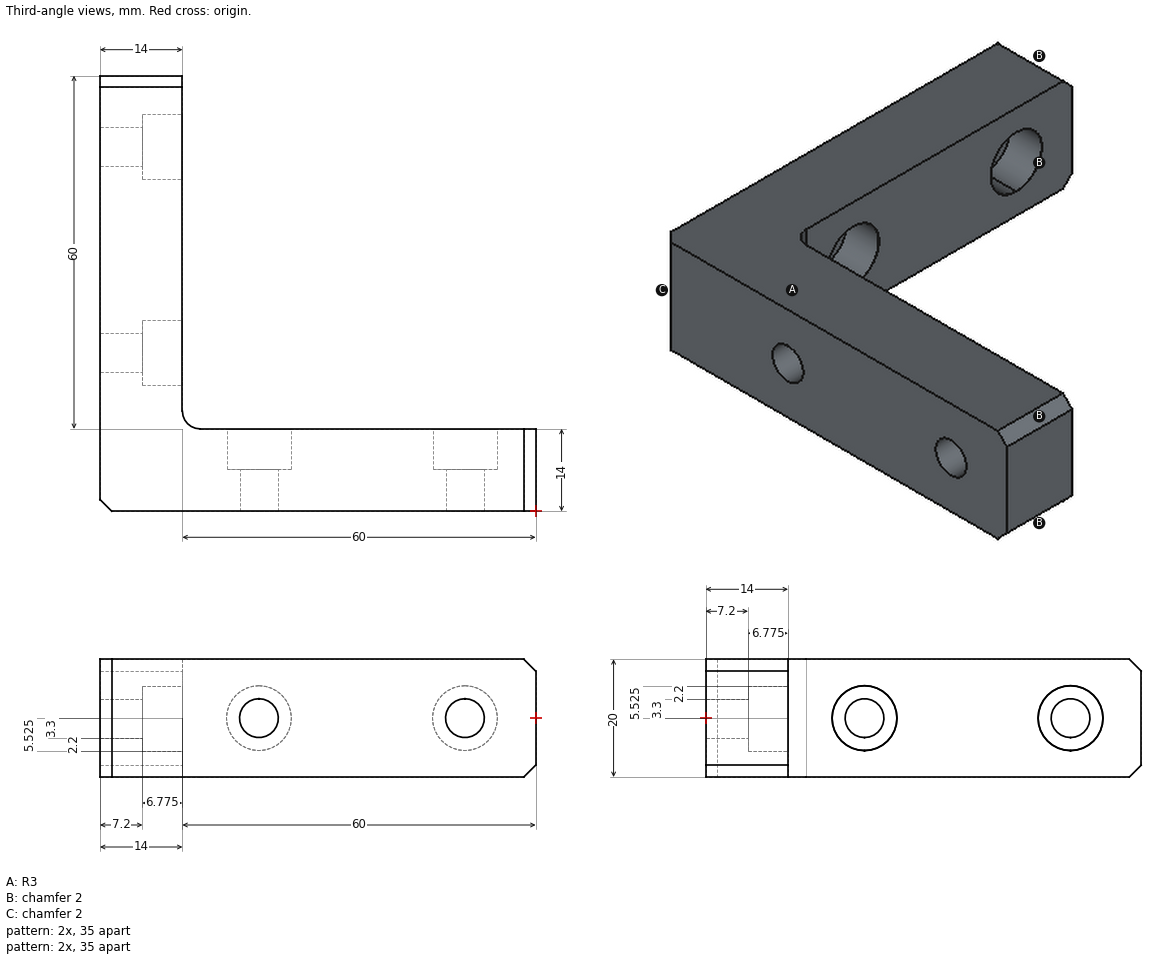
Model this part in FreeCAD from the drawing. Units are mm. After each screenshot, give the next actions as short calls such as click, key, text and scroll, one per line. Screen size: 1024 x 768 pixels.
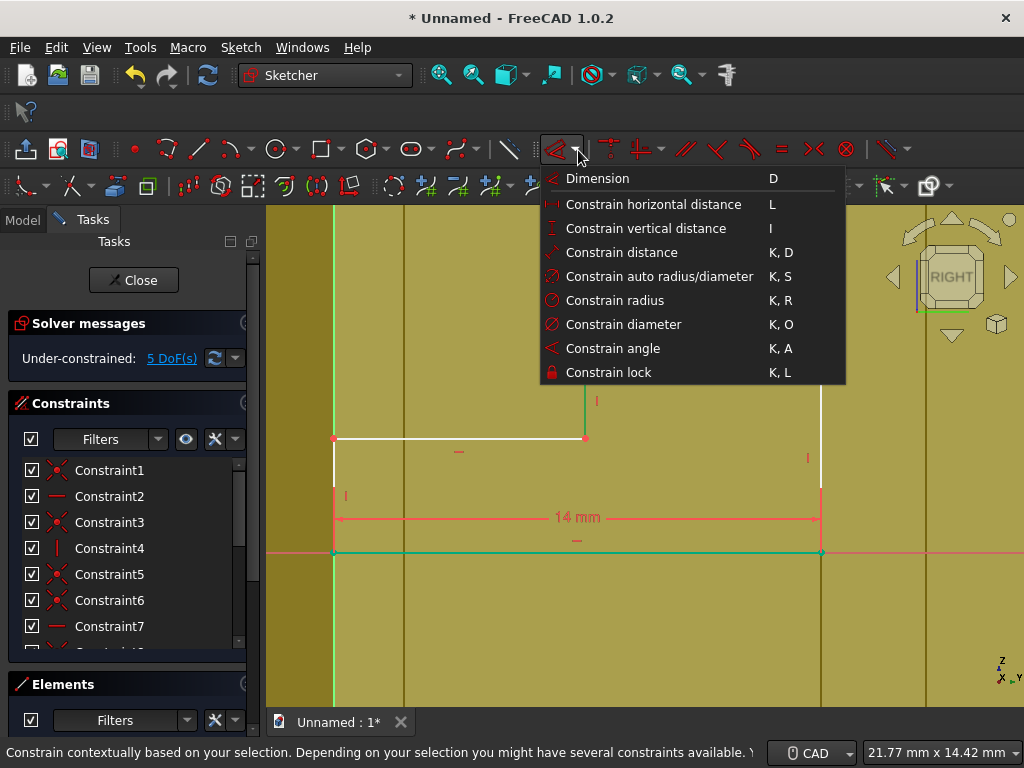
click(693, 228)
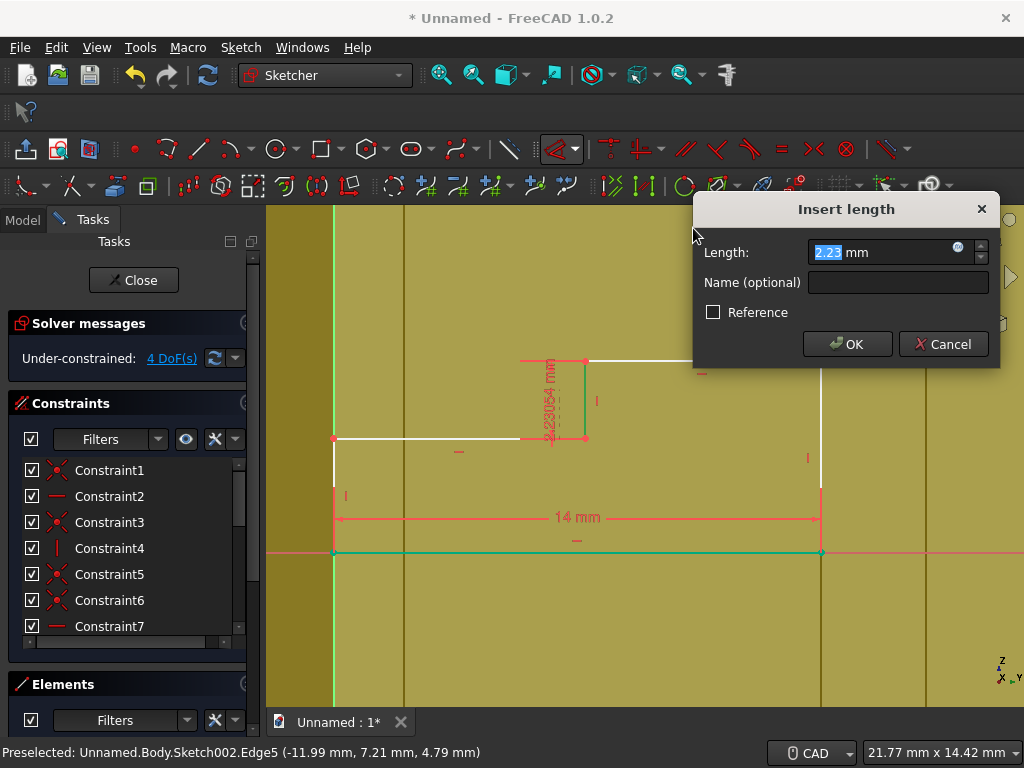
text(2.2)
key(Return)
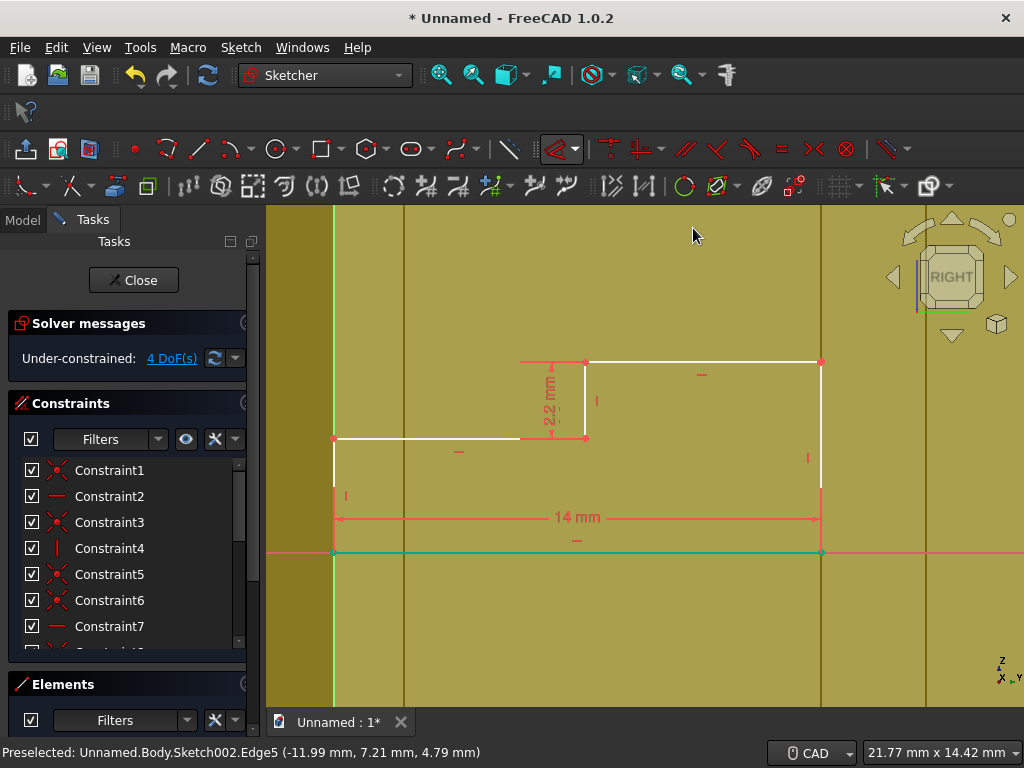
click(510, 439)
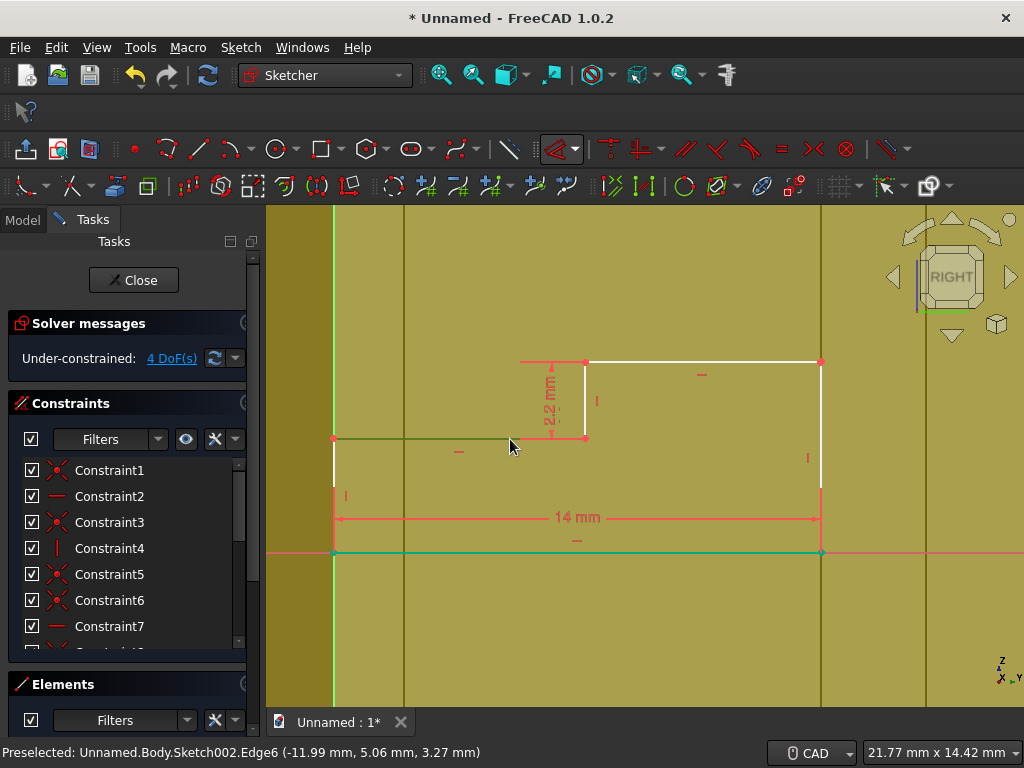
key(l)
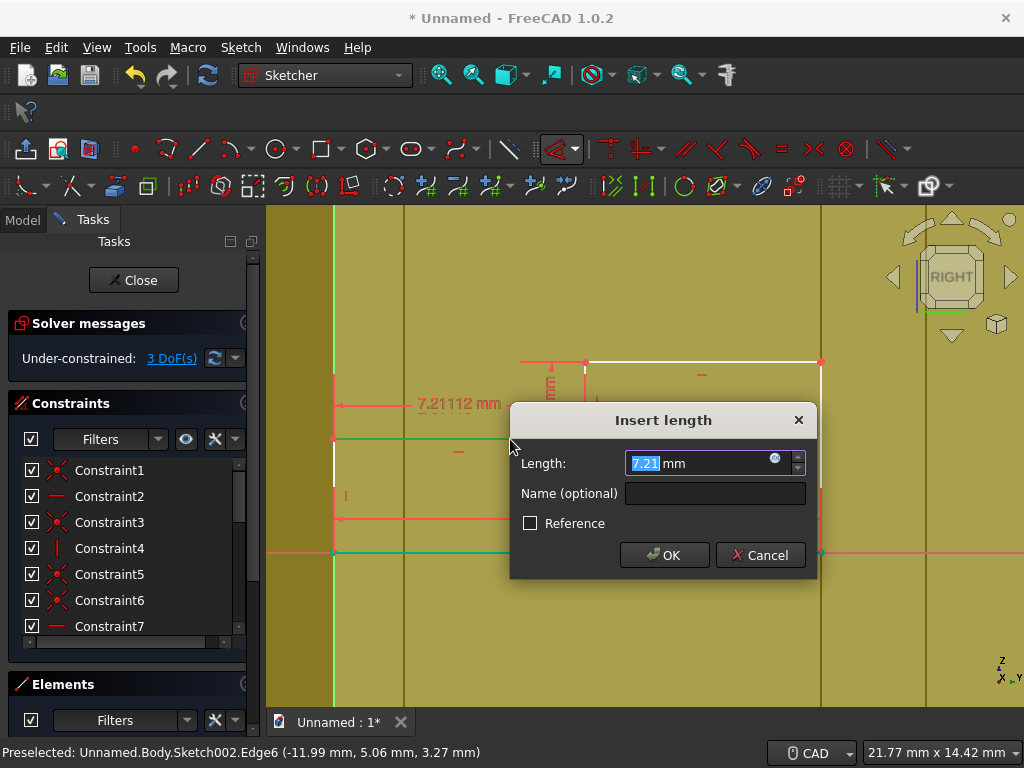
text(7.2)
key(Return)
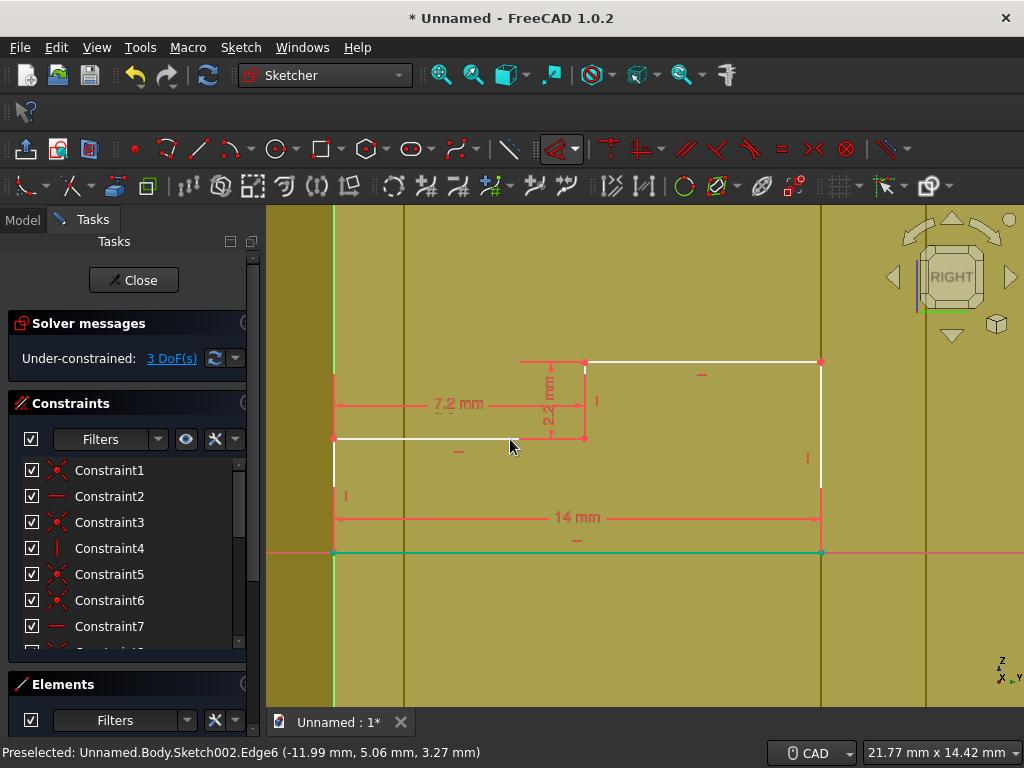
click(334, 473)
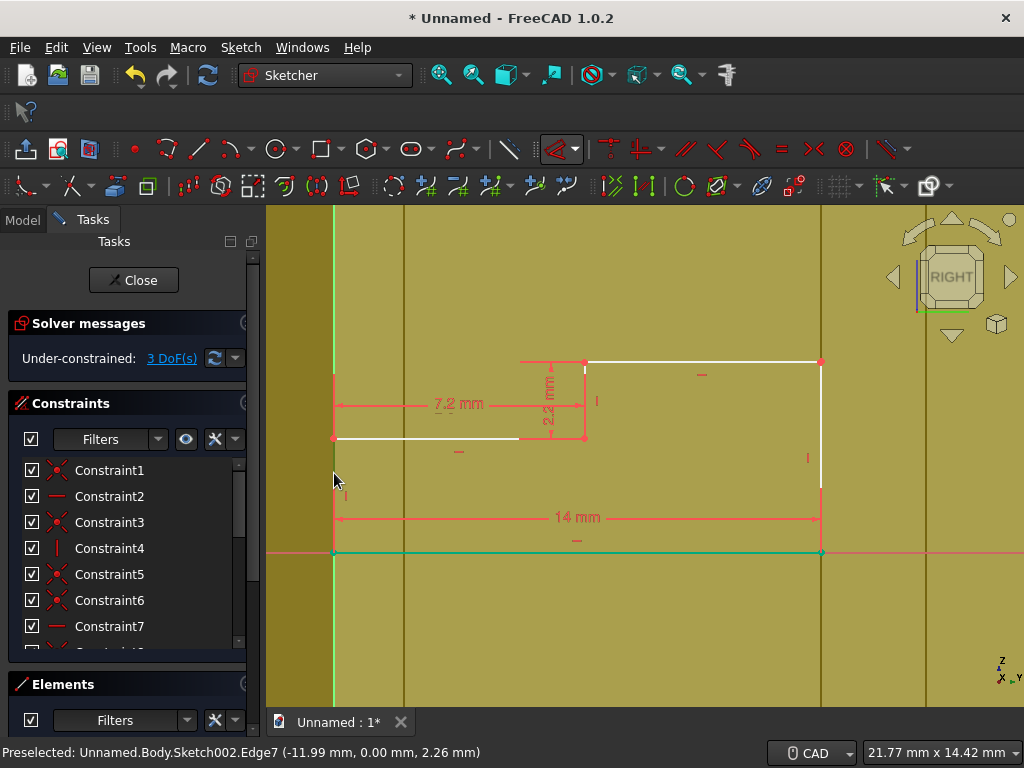
click(578, 150)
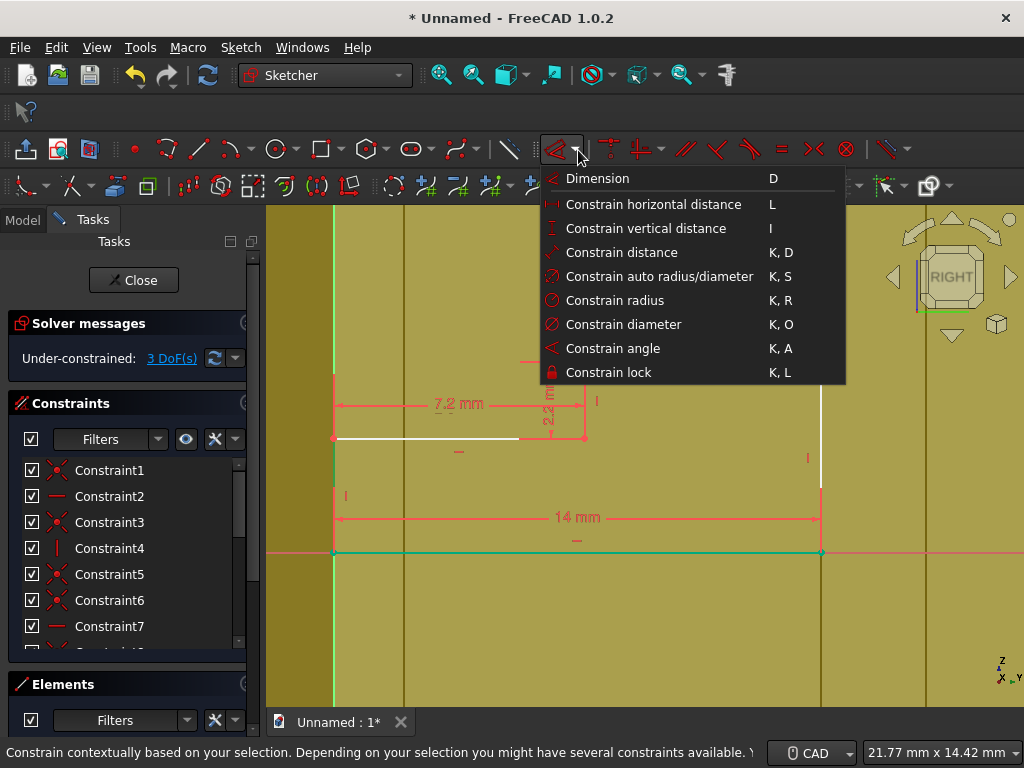
click(693, 228)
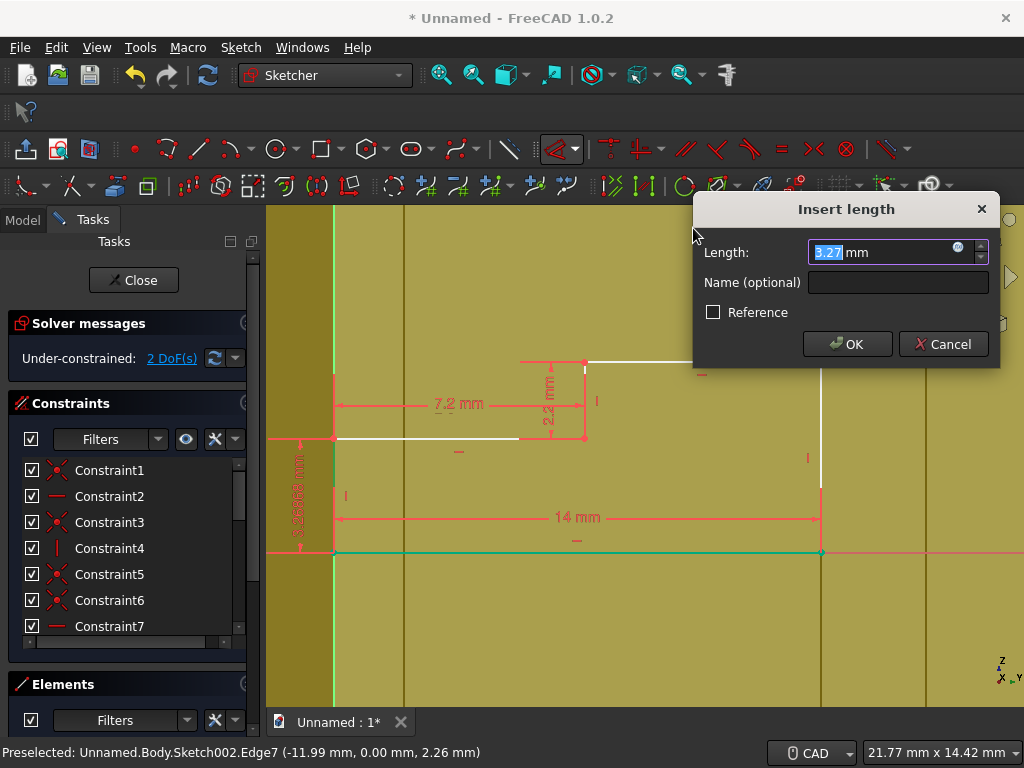
text(3.3)
key(Return)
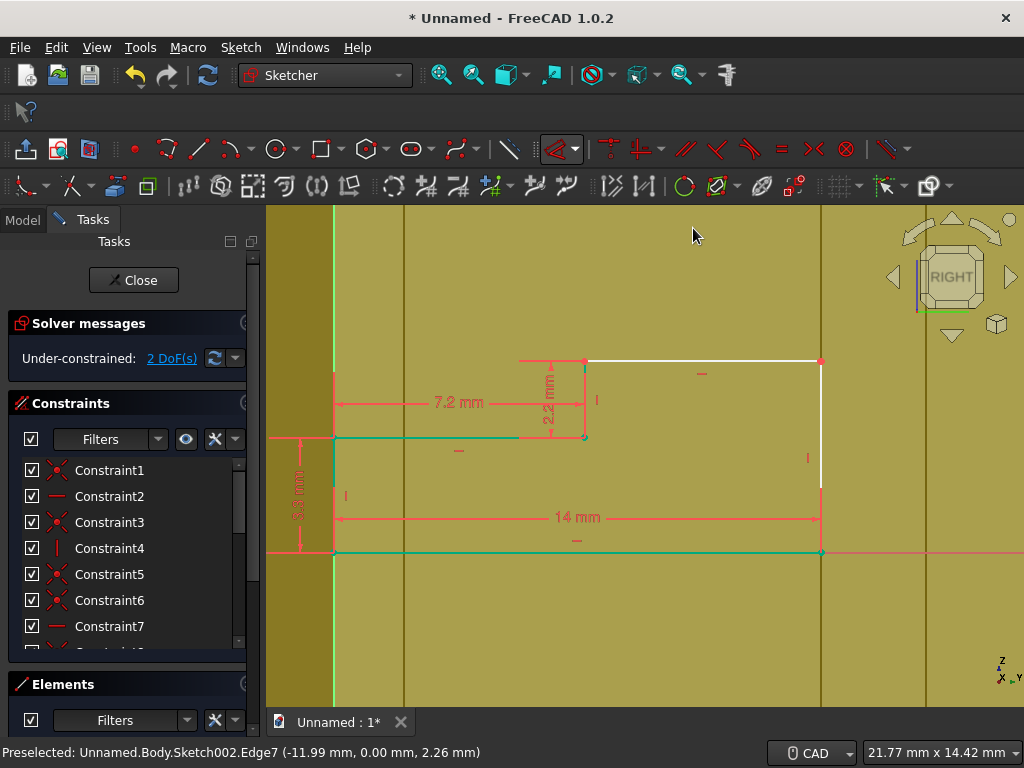
click(821, 495)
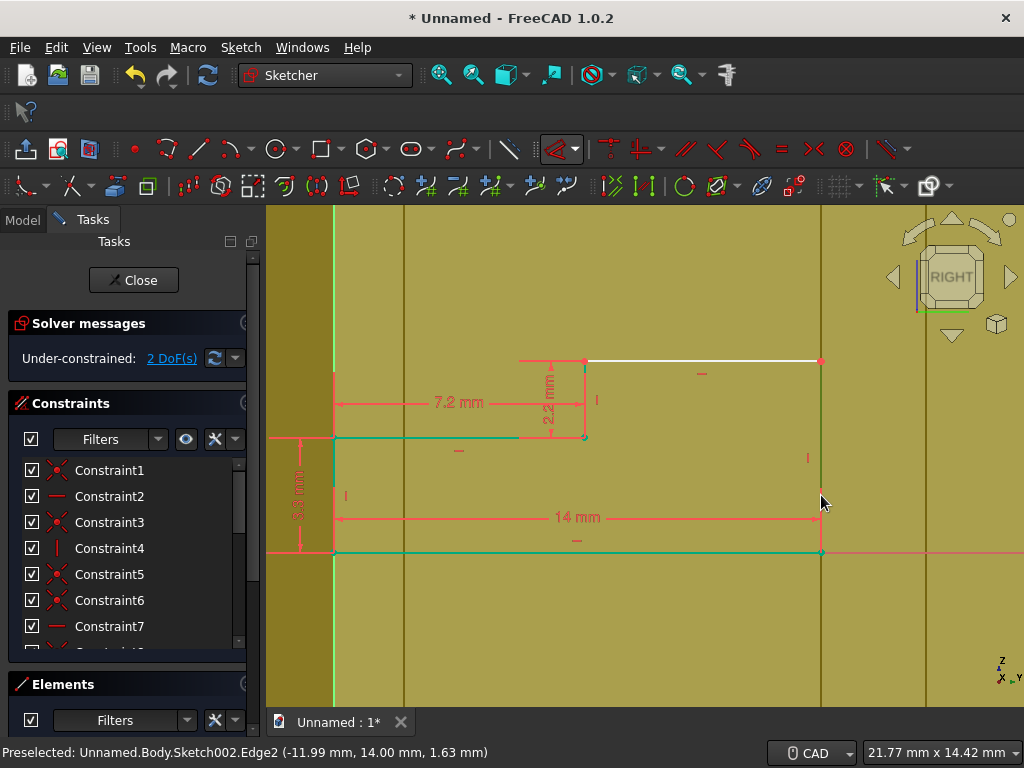
click(578, 150)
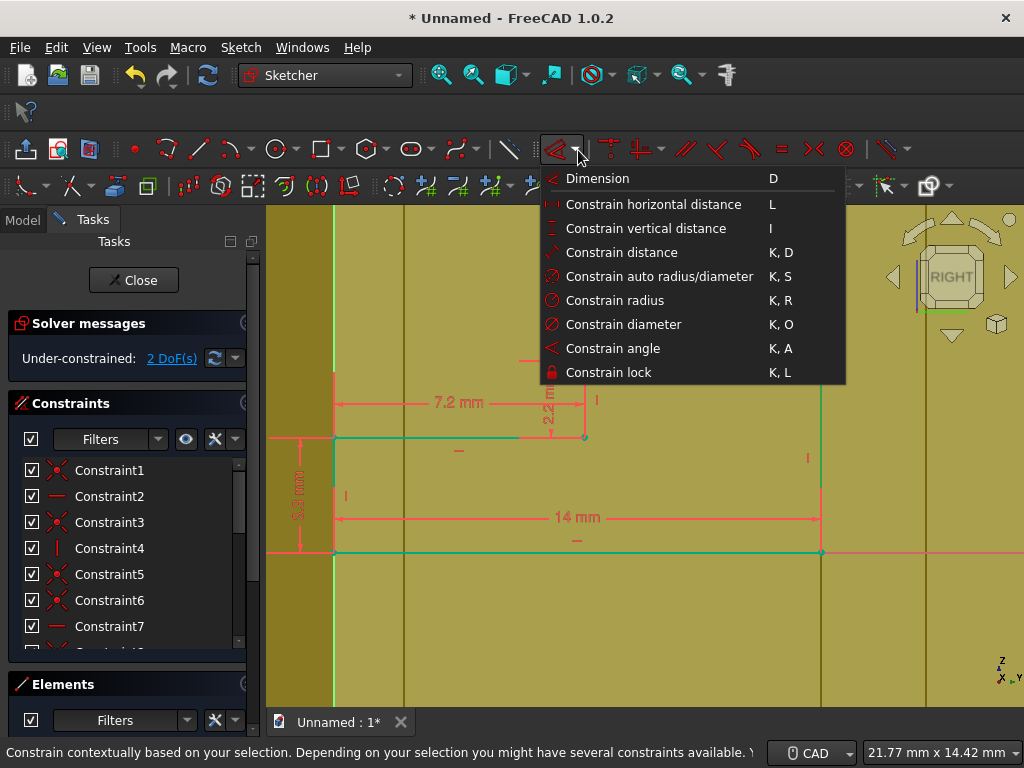
click(693, 228)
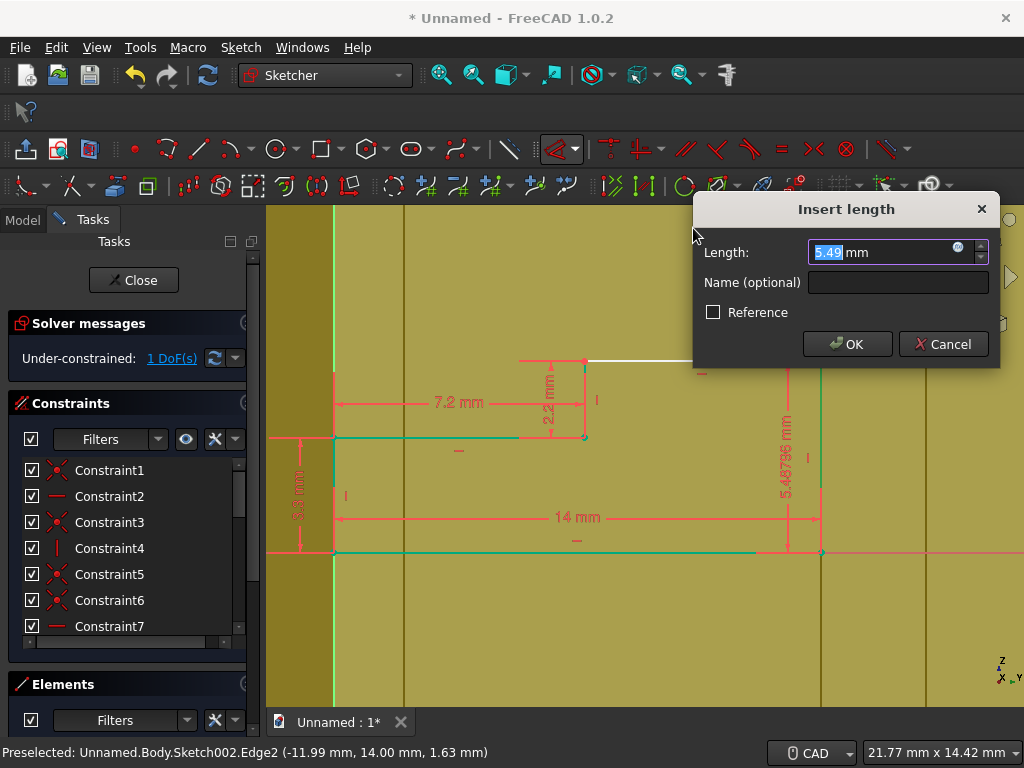
text(5.525)
key(Return)